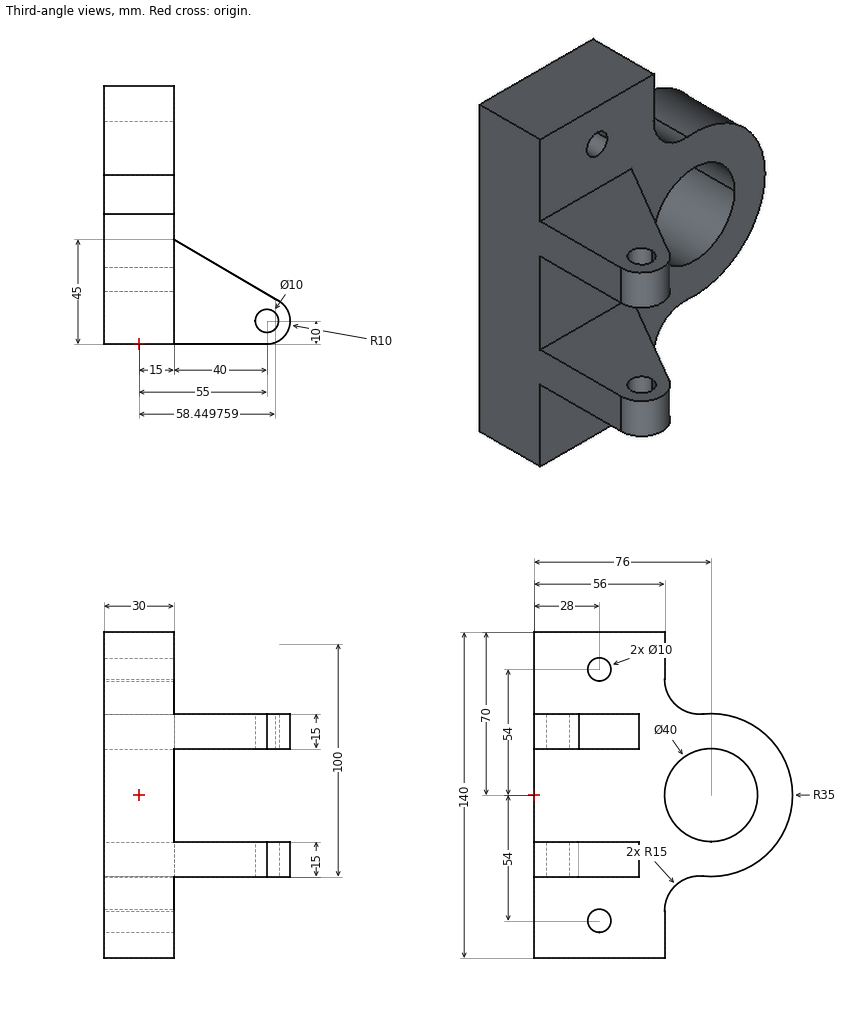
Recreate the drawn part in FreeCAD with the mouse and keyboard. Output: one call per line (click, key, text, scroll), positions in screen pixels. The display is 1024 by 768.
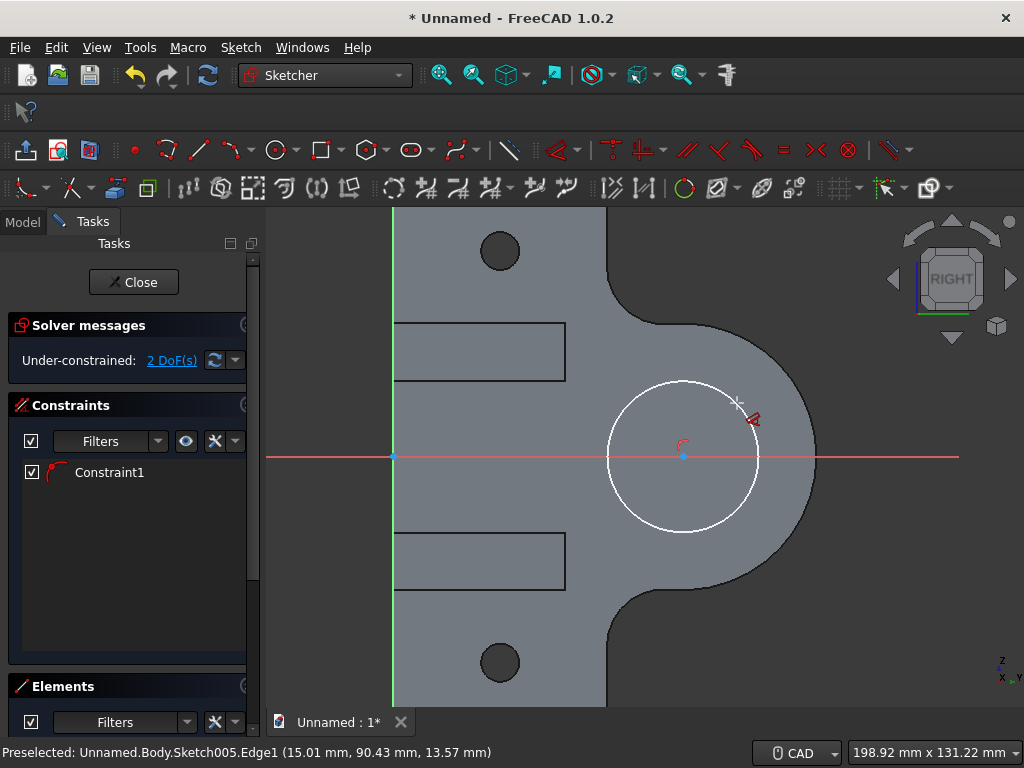
click(736, 403)
click(758, 380)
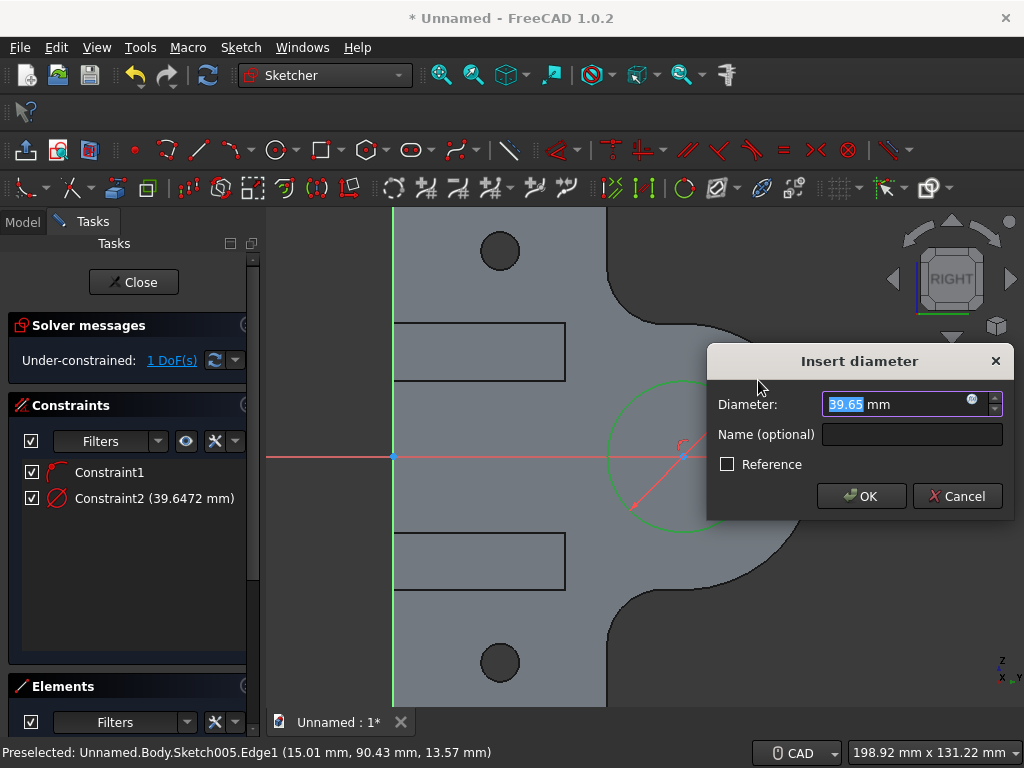
text(40)
key(Return)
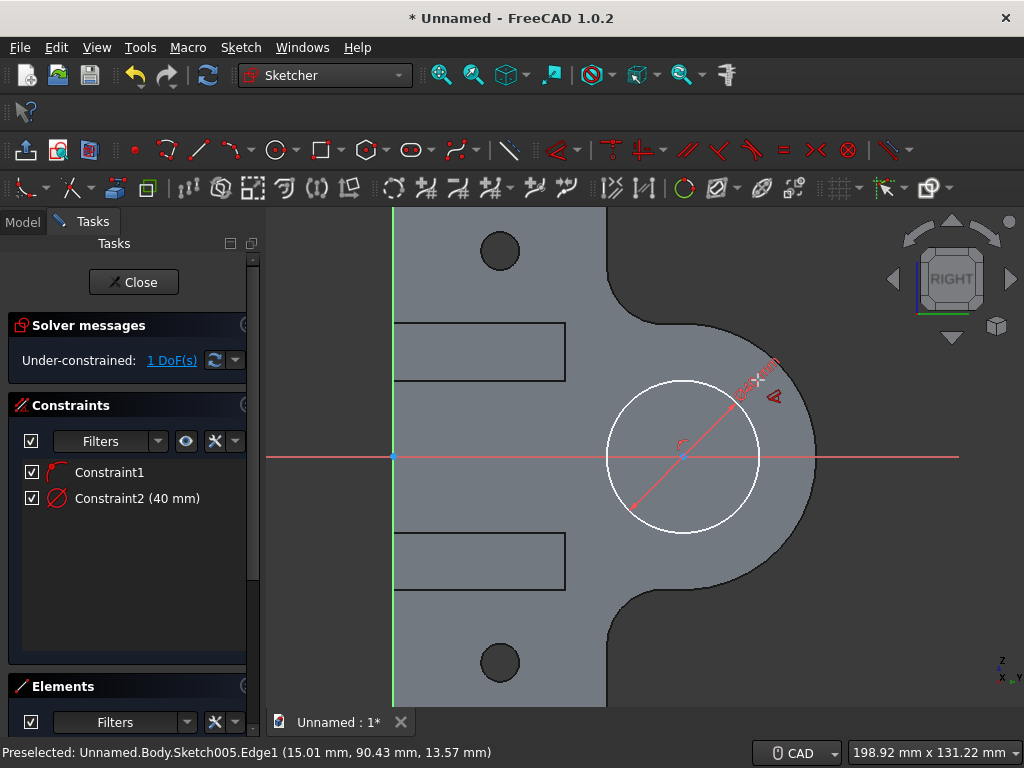
click(683, 457)
click(538, 423)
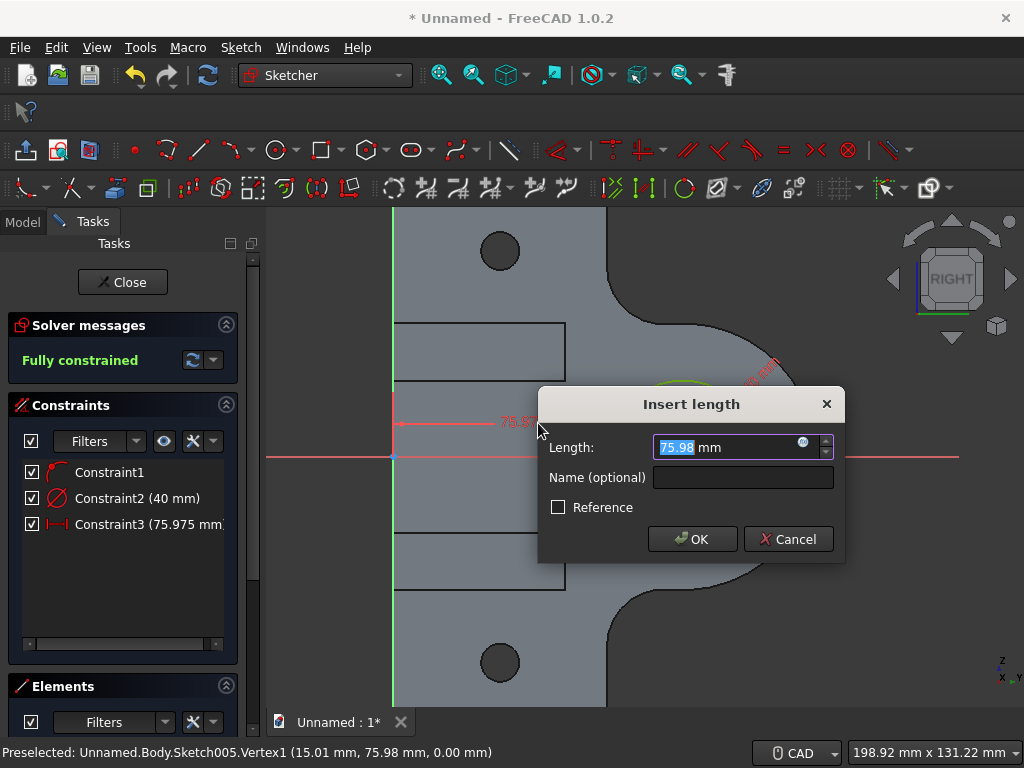
text(76)
key(Return)
key(Escape)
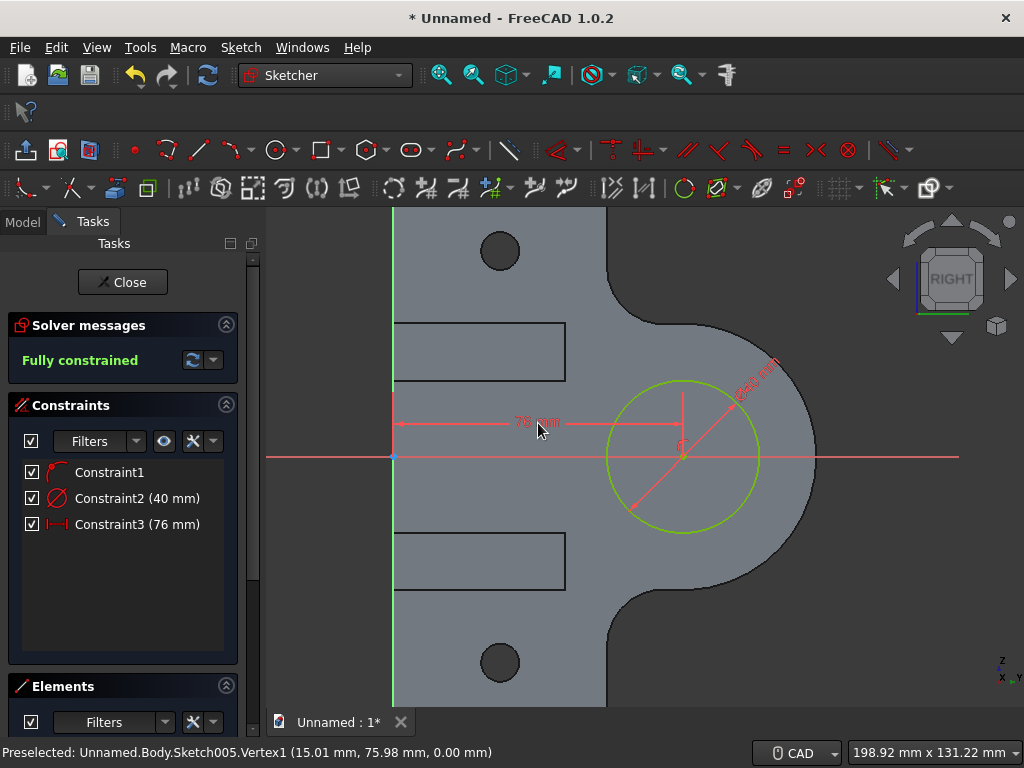
click(123, 282)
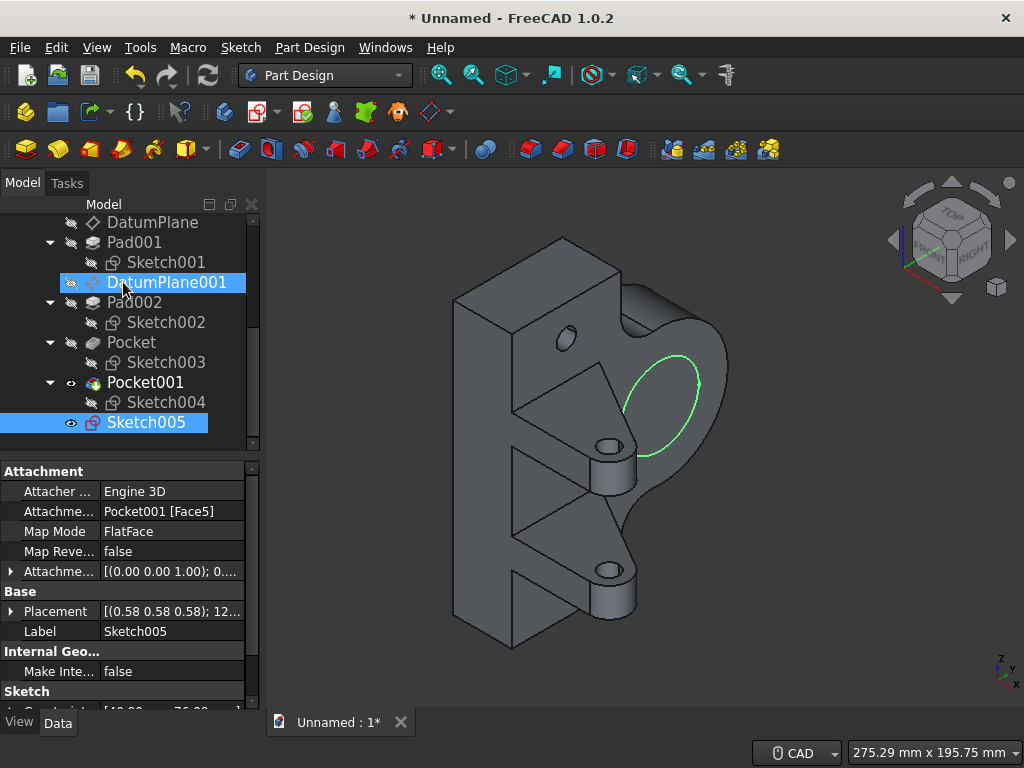
click(240, 150)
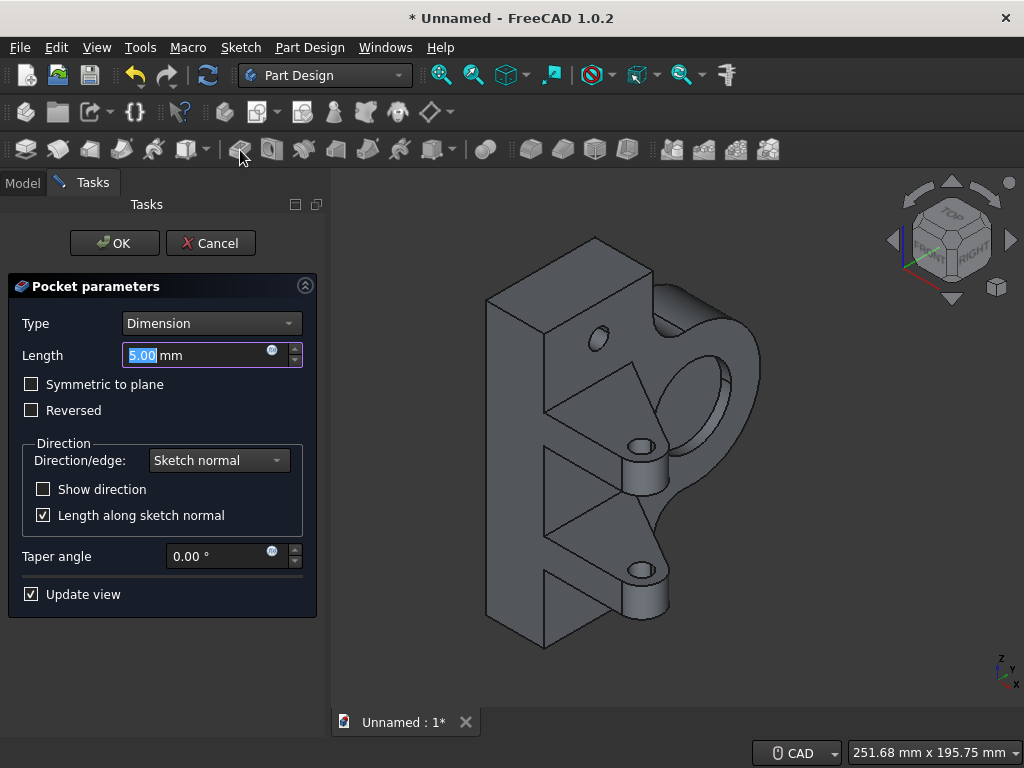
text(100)
key(Tab)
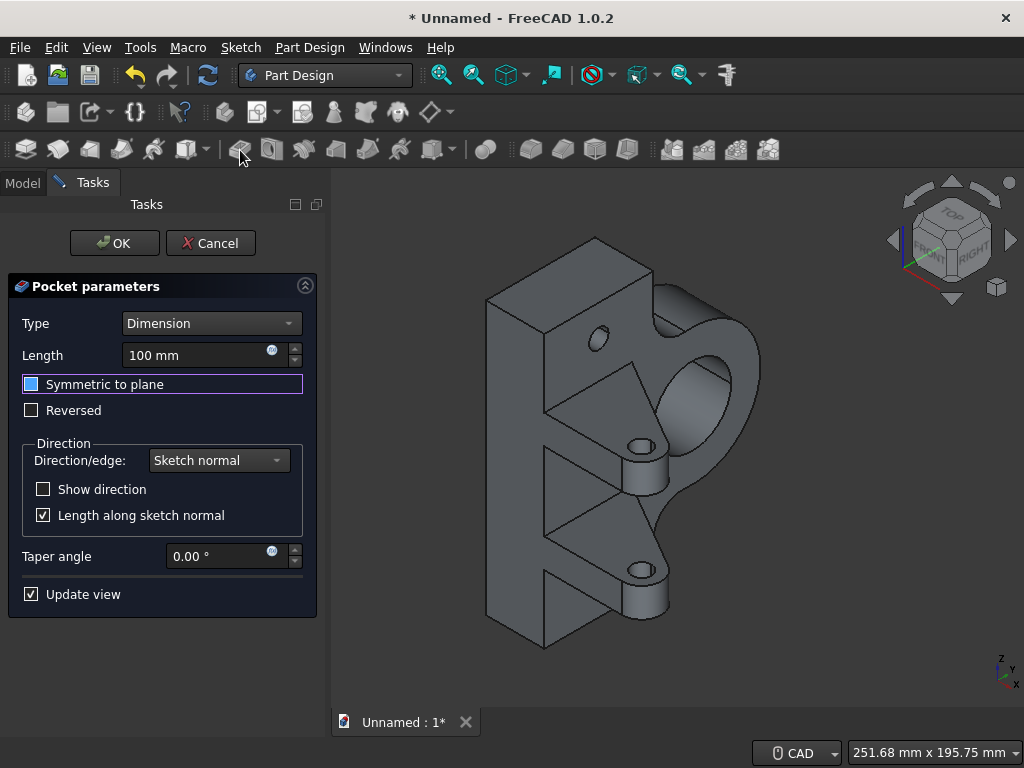
click(115, 243)